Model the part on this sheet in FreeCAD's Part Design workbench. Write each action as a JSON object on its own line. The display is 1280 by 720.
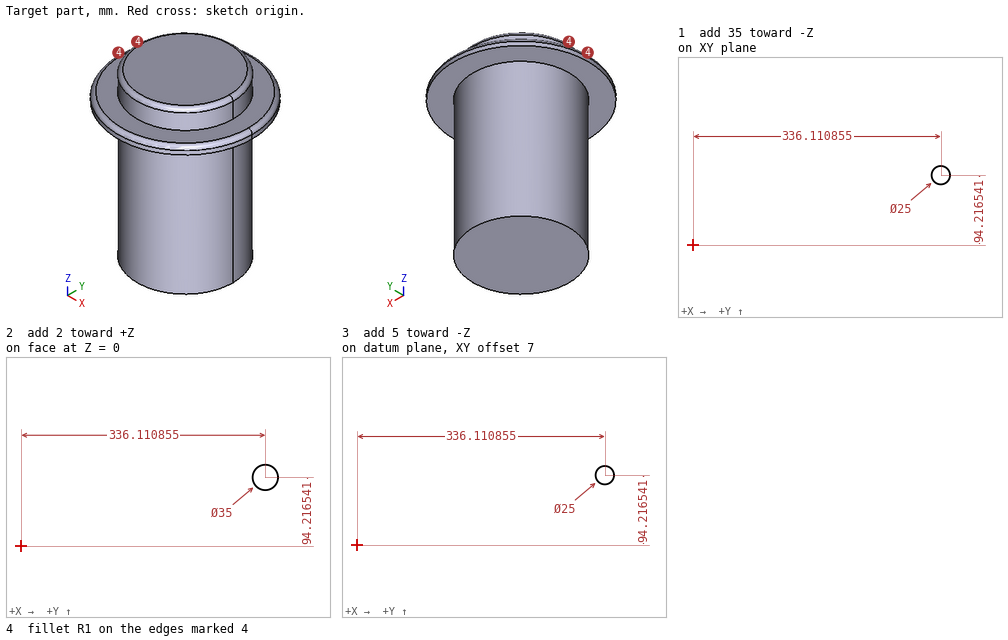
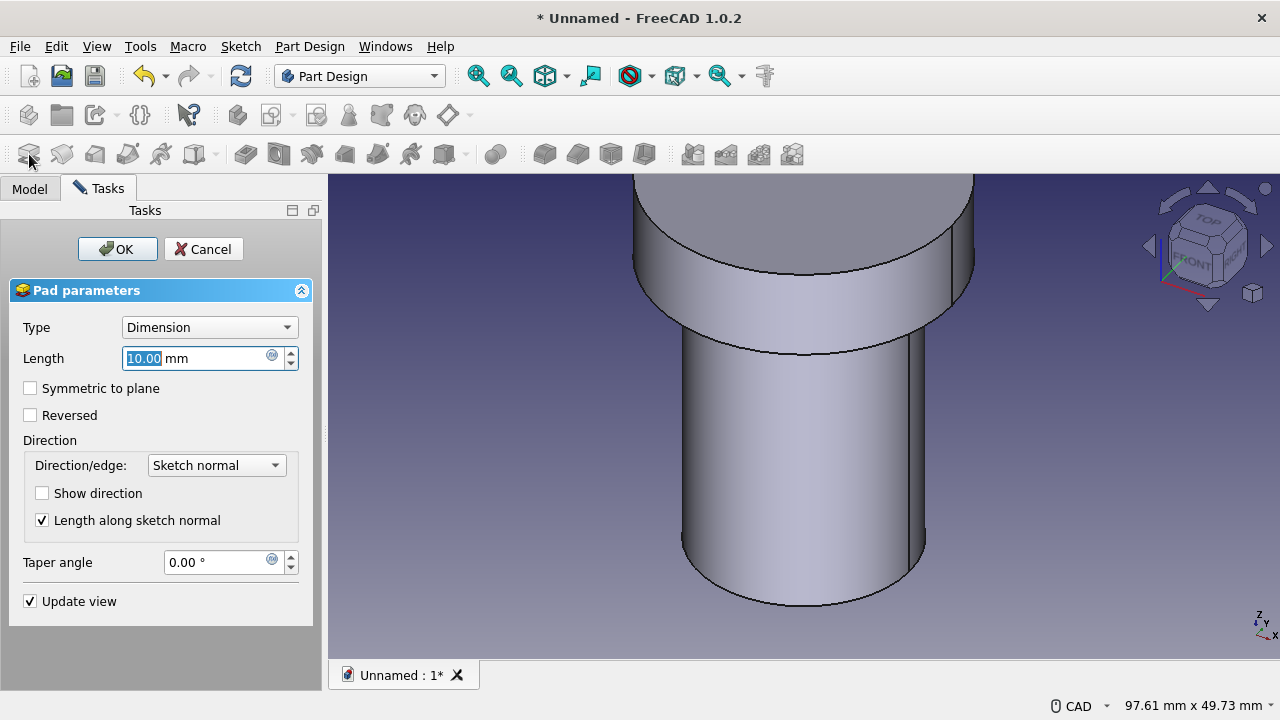
{"action": "type", "text": "2"}
{"action": "key", "text": "Tab"}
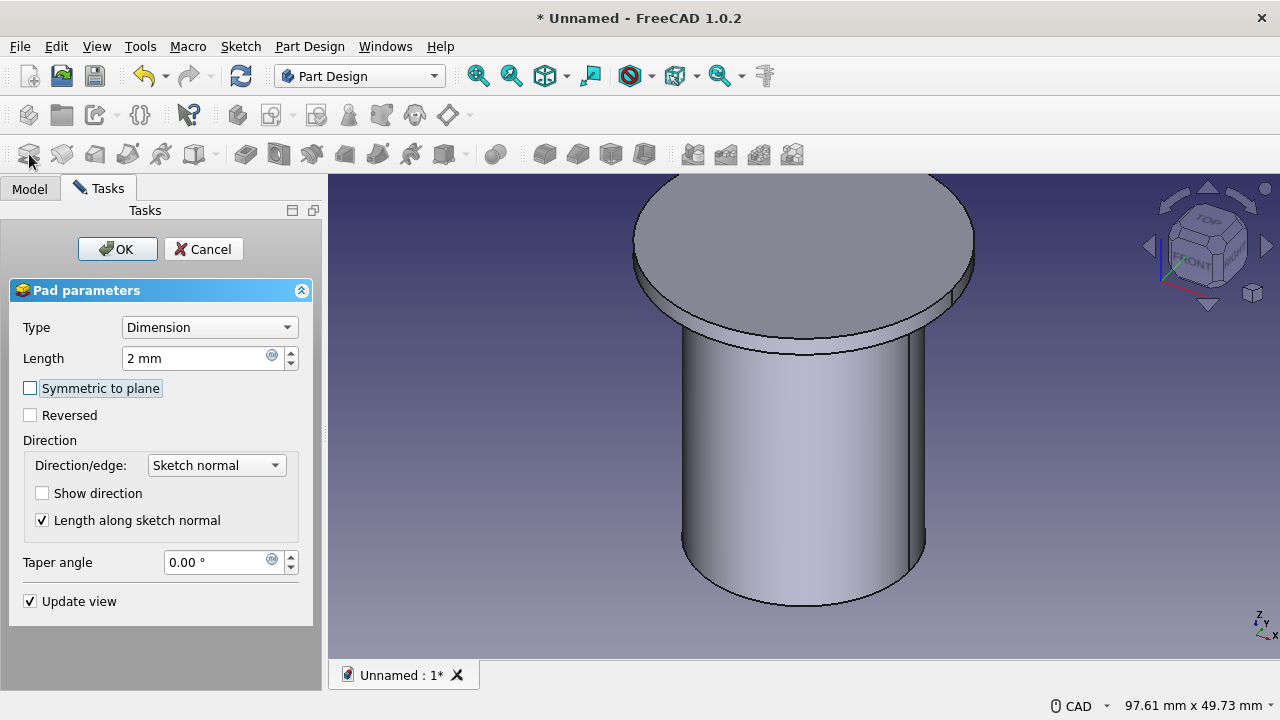
{"action": "left_click", "coordinate": [118, 249]}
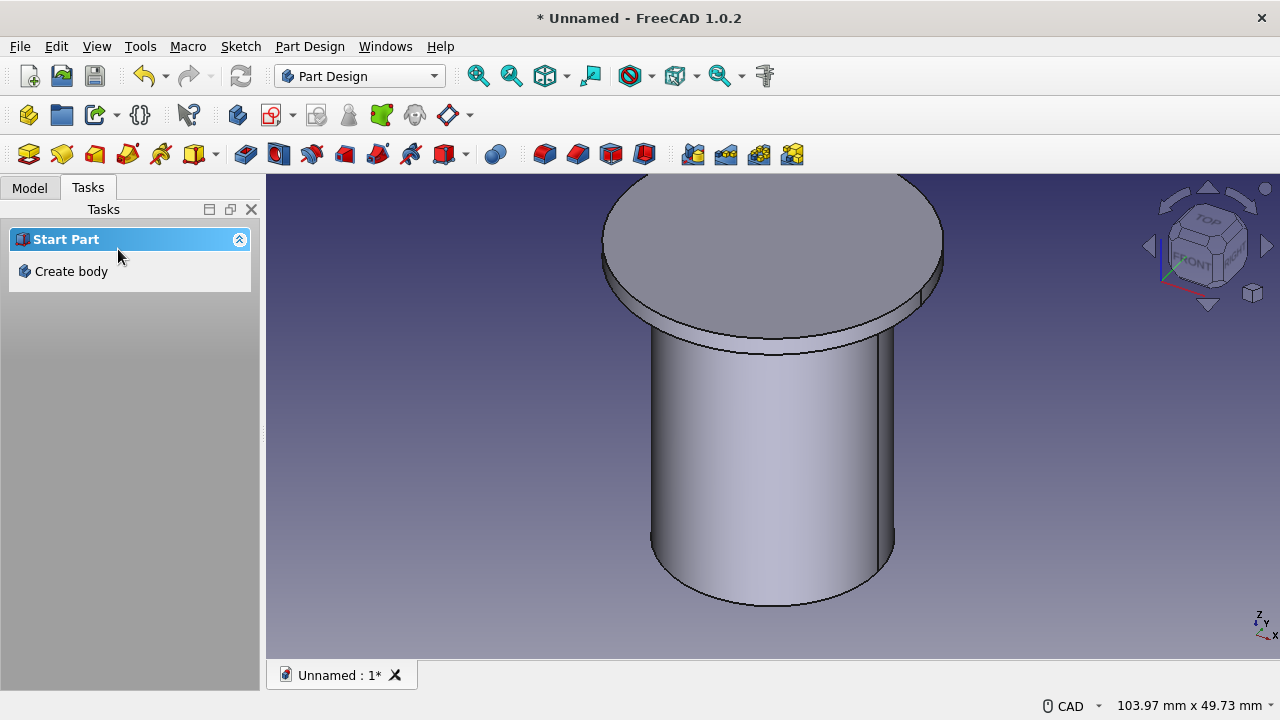
{"action": "left_click", "coordinate": [479, 76]}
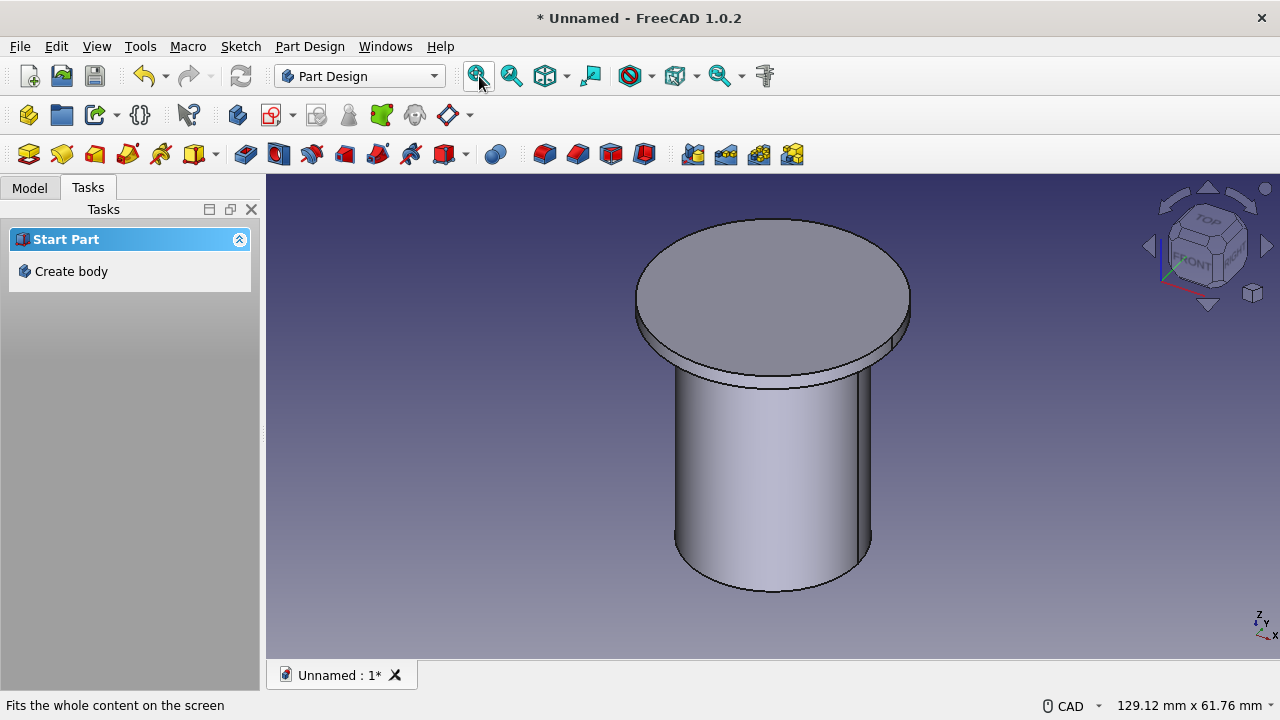
{"action": "left_click", "coordinate": [30, 188]}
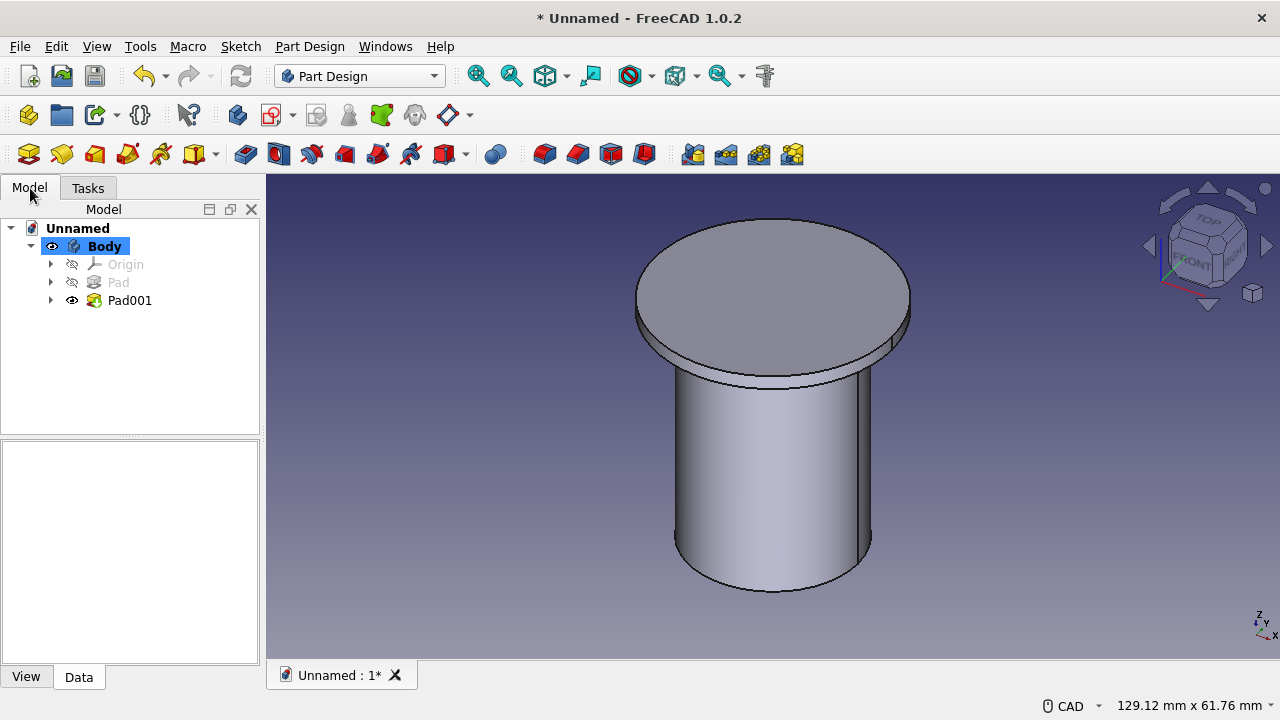
{"action": "left_click", "coordinate": [51, 264]}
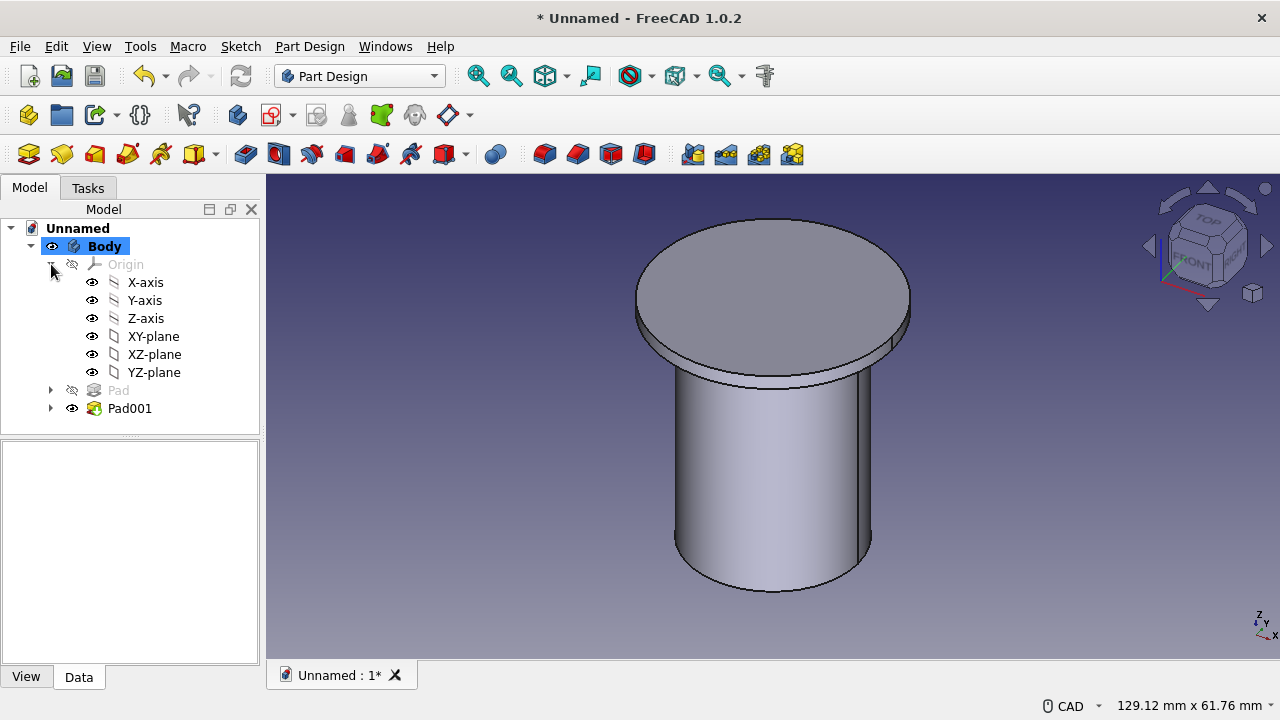
{"action": "left_click", "coordinate": [137, 336]}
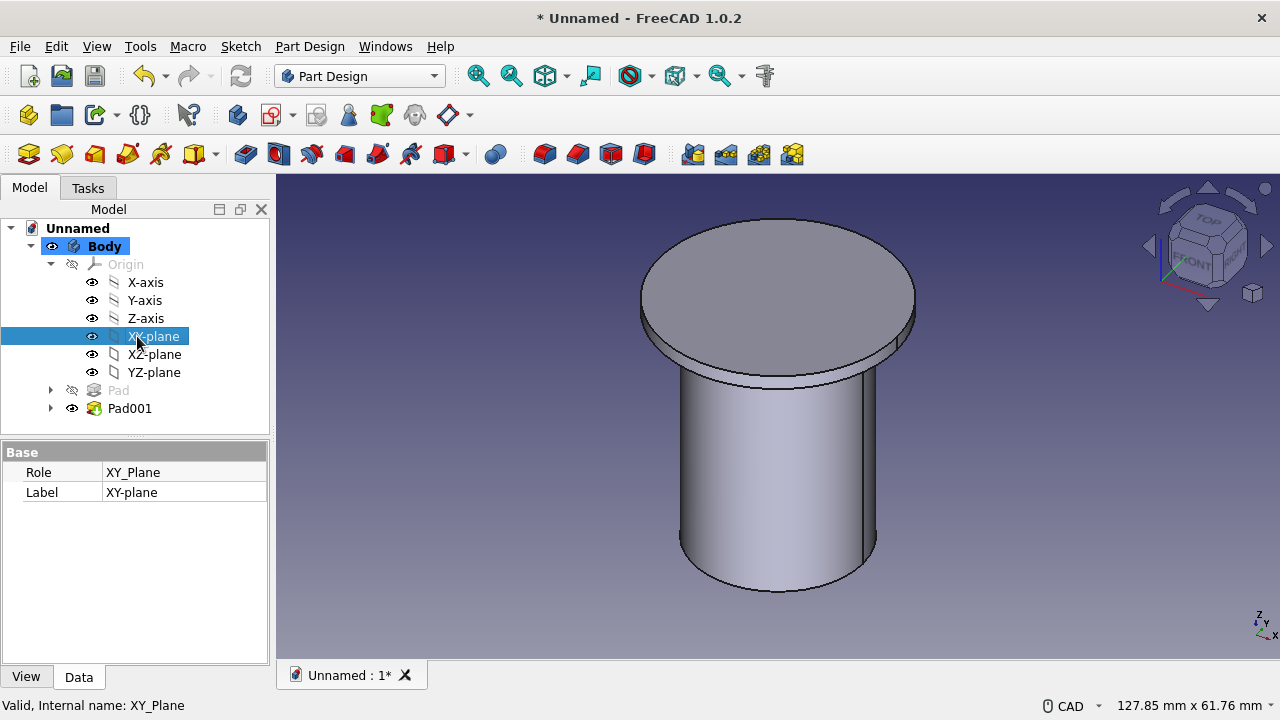
{"action": "left_click", "coordinate": [448, 116]}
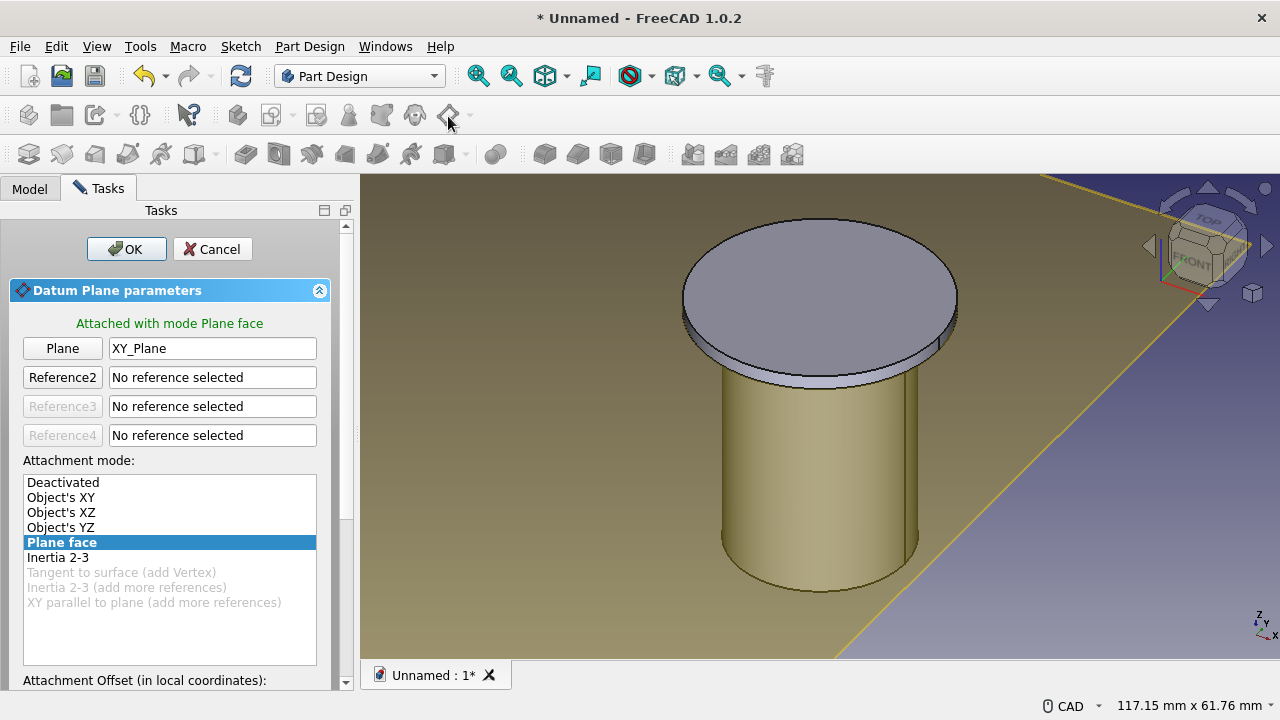
{"action": "scroll", "coordinate": [346, 455], "scroll_direction": "down", "scroll_amount": 3}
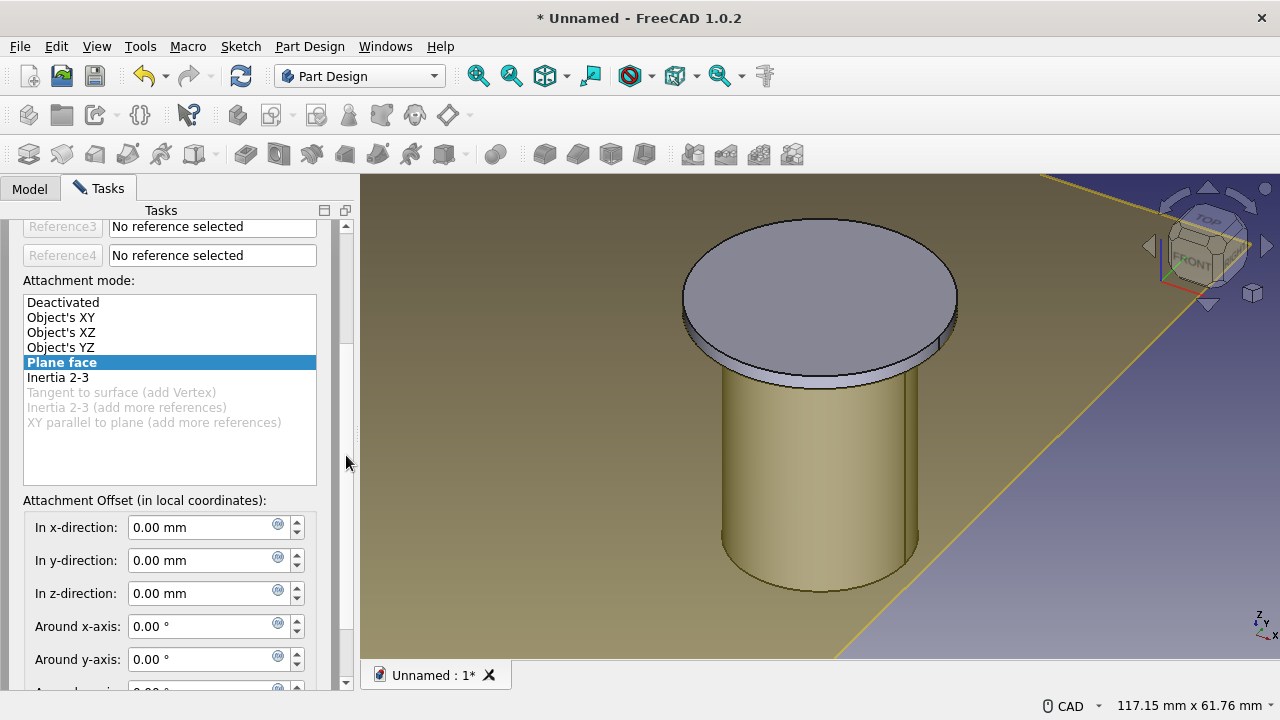
{"action": "triple_click", "coordinate": [210, 594]}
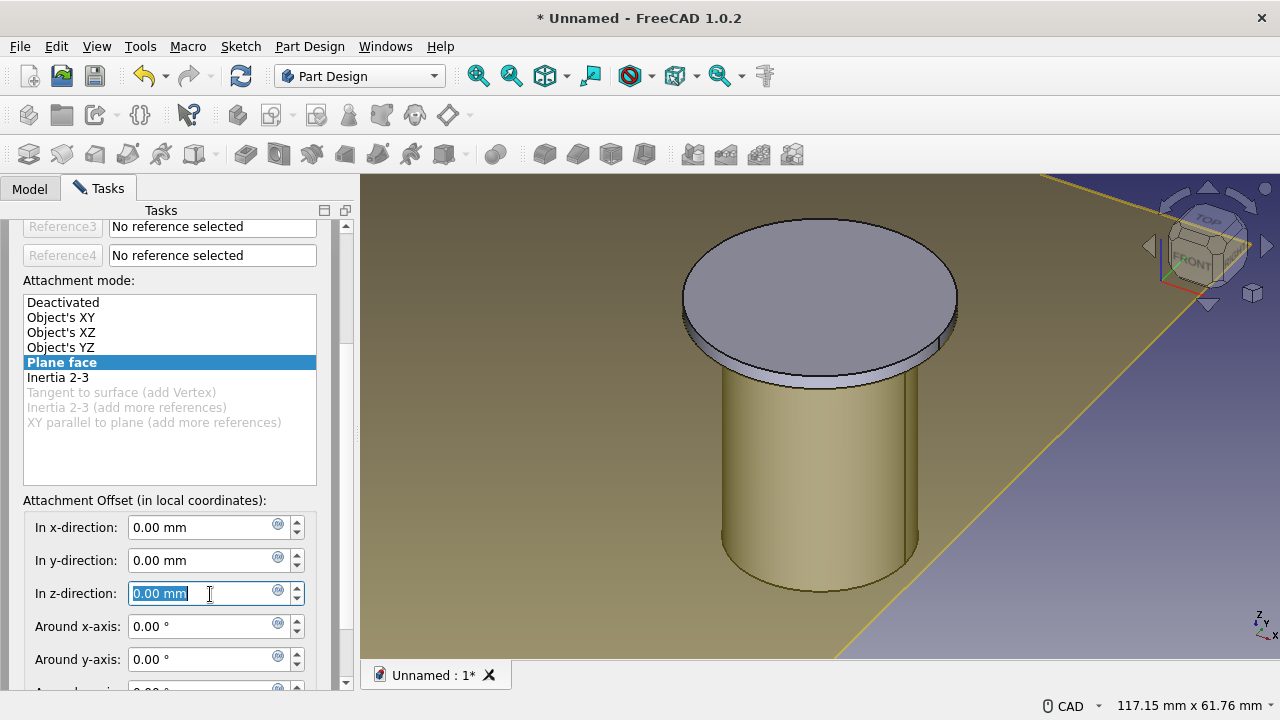
{"action": "type", "text": "7"}
{"action": "key", "text": "Tab"}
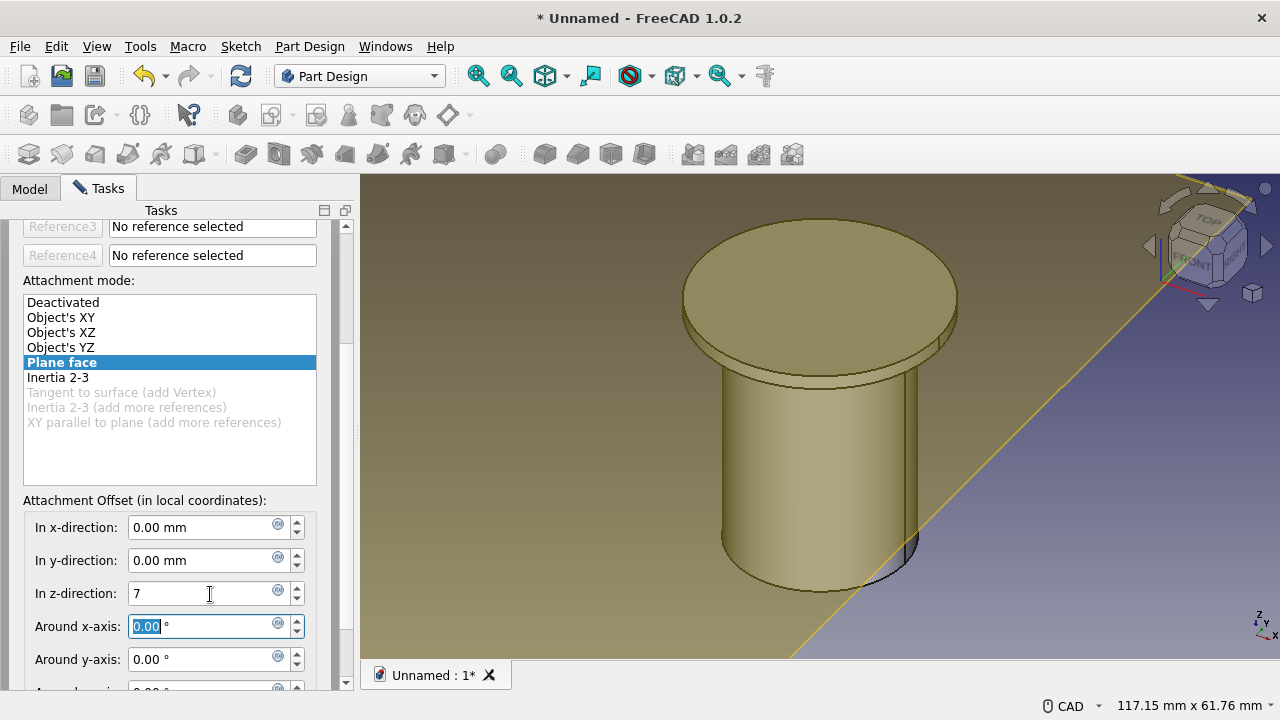
{"action": "scroll", "coordinate": [346, 455], "scroll_direction": "up", "scroll_amount": 4}